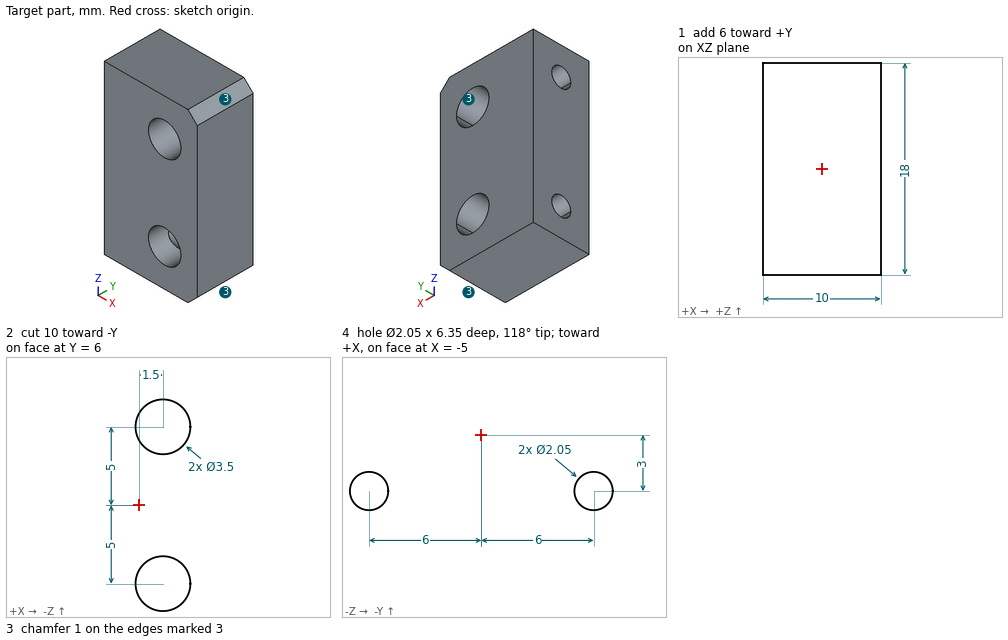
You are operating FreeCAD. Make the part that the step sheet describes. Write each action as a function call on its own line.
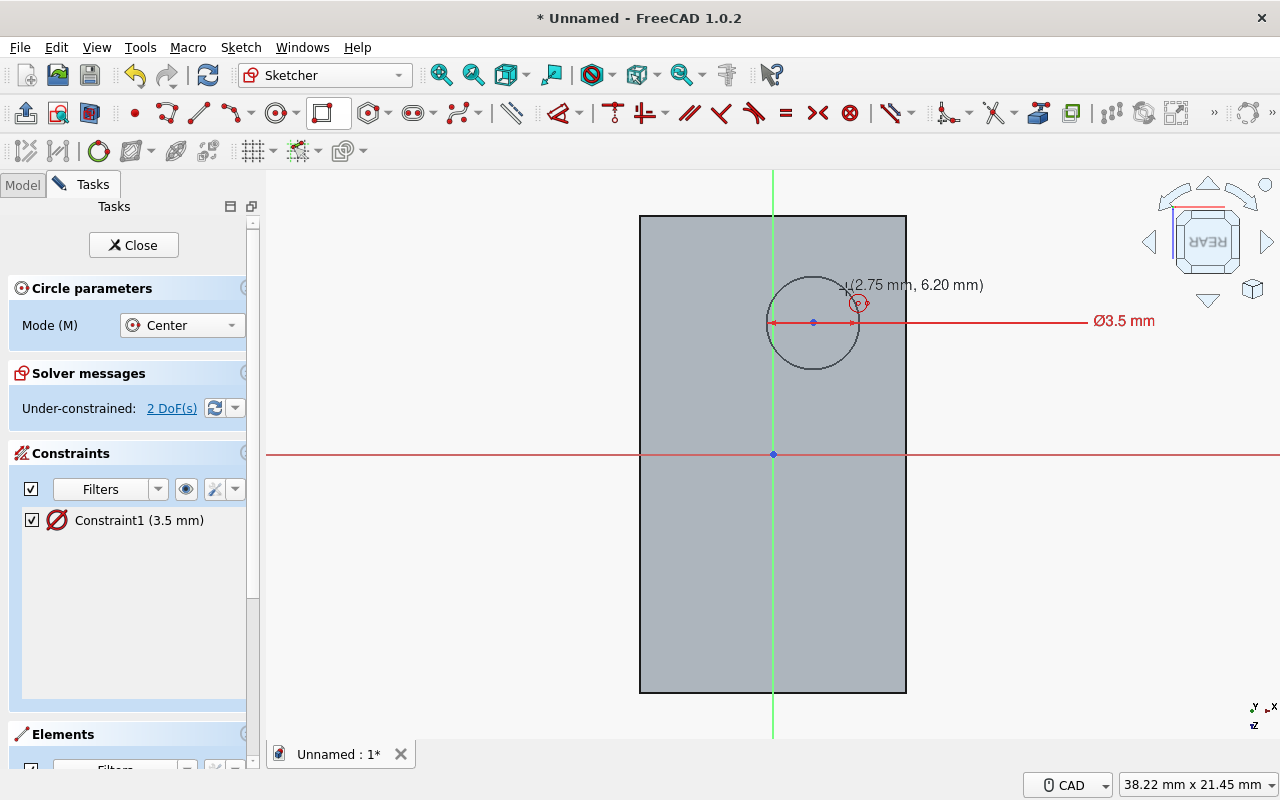
click(813, 587)
move(846, 554)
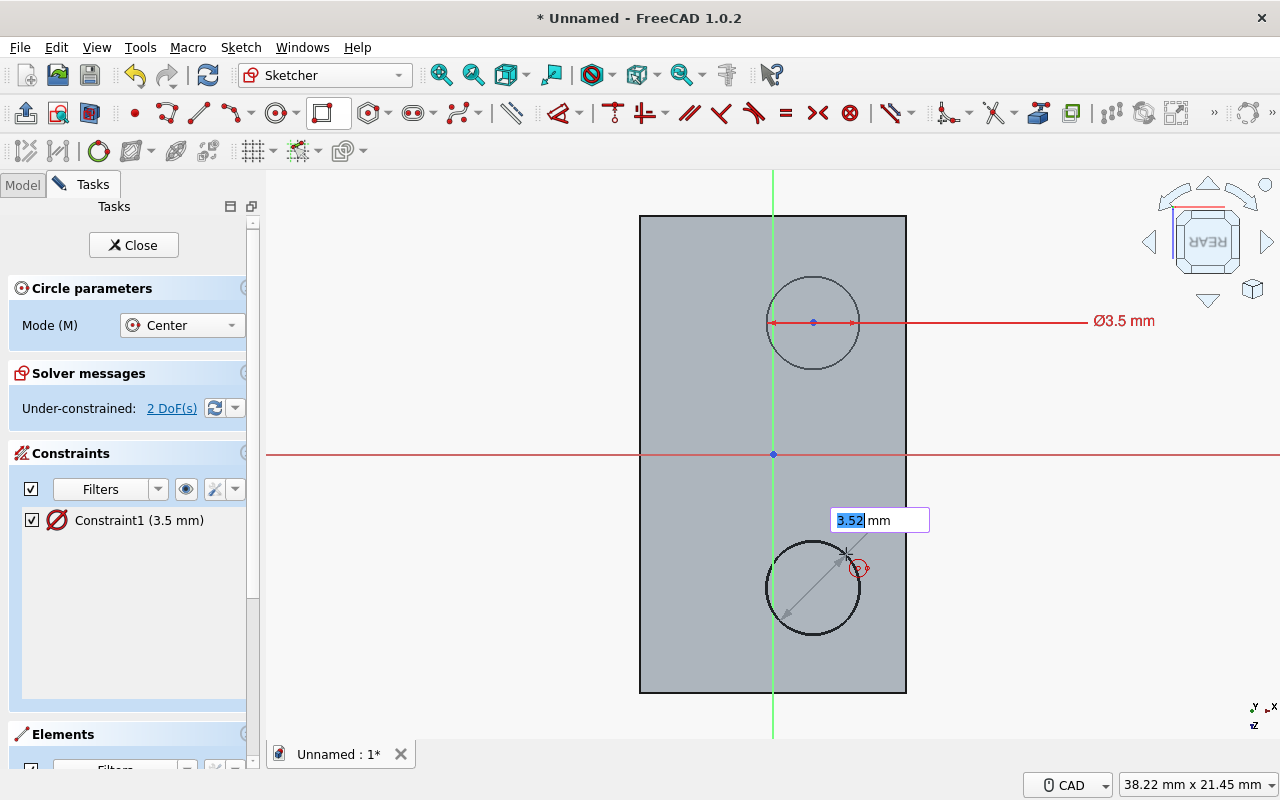
text(3.5)
key(Return)
key(Escape)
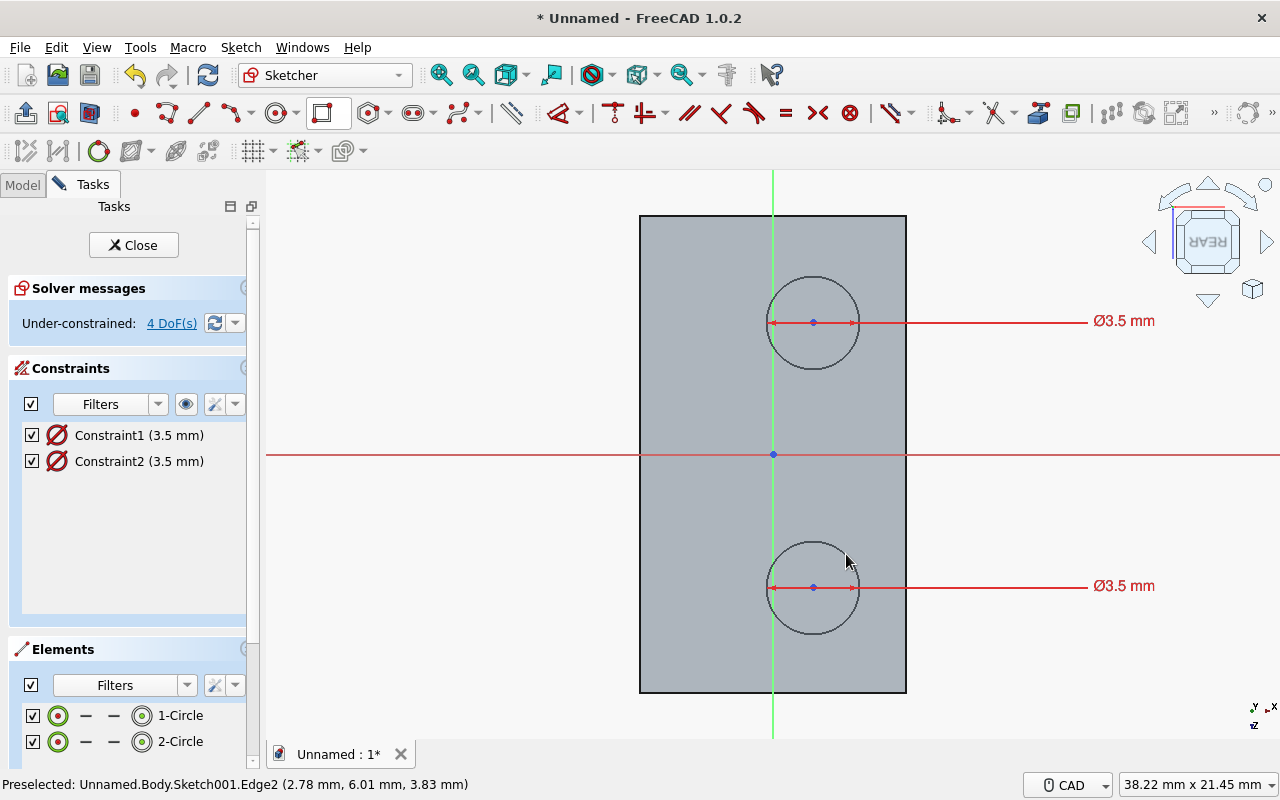
click(813, 323)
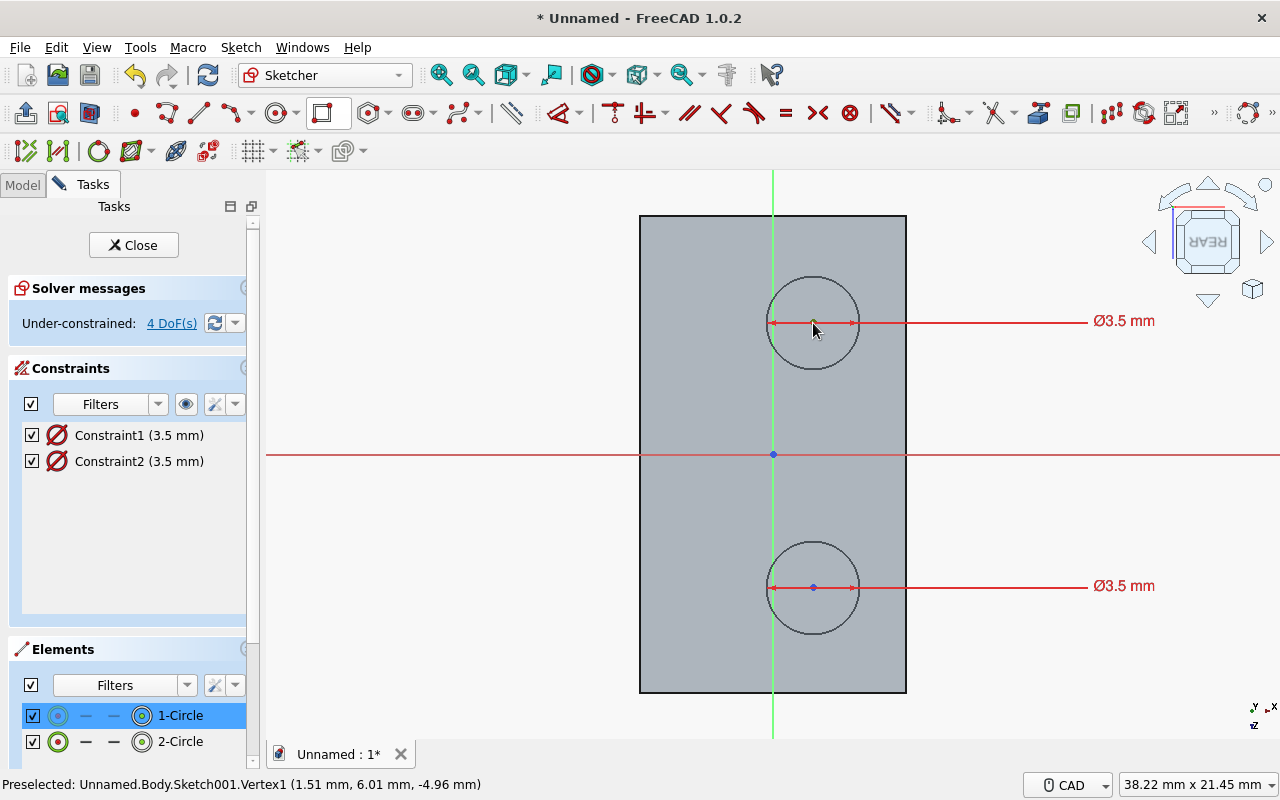
click(813, 588)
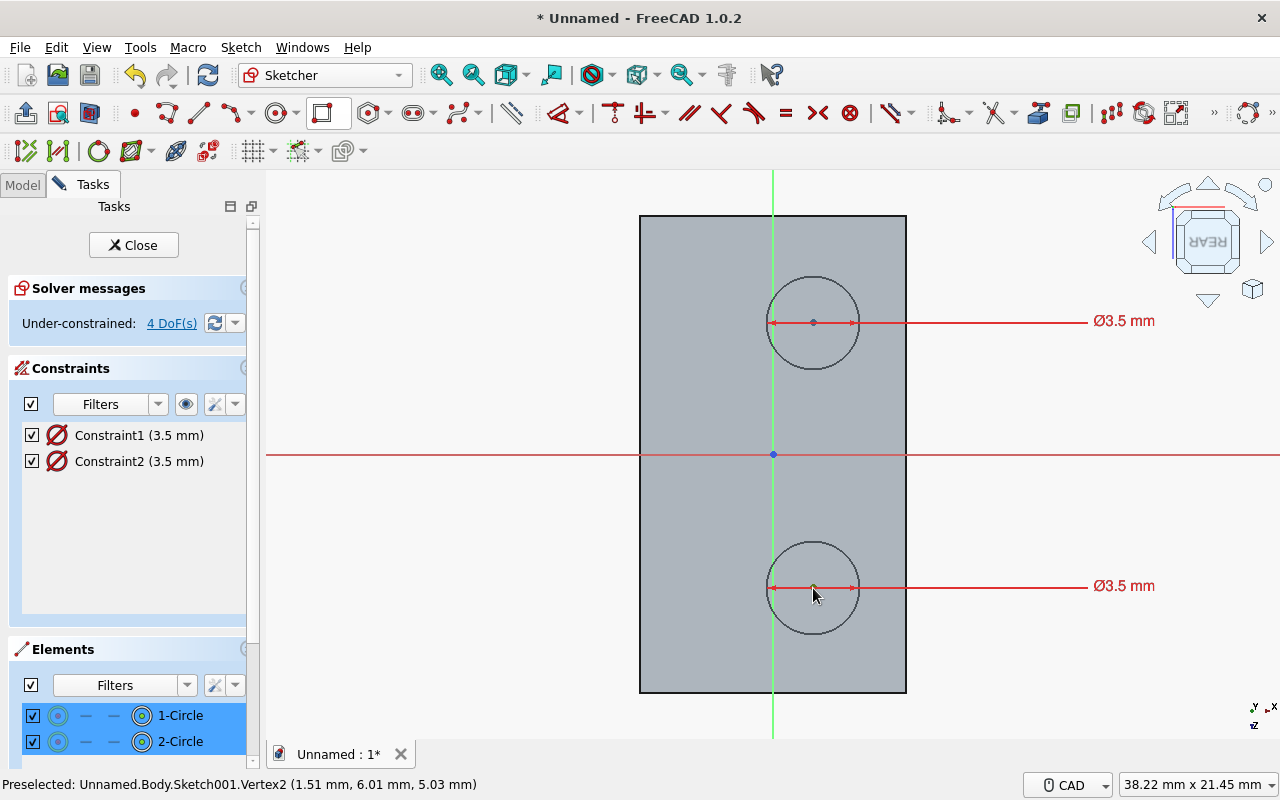
key(v)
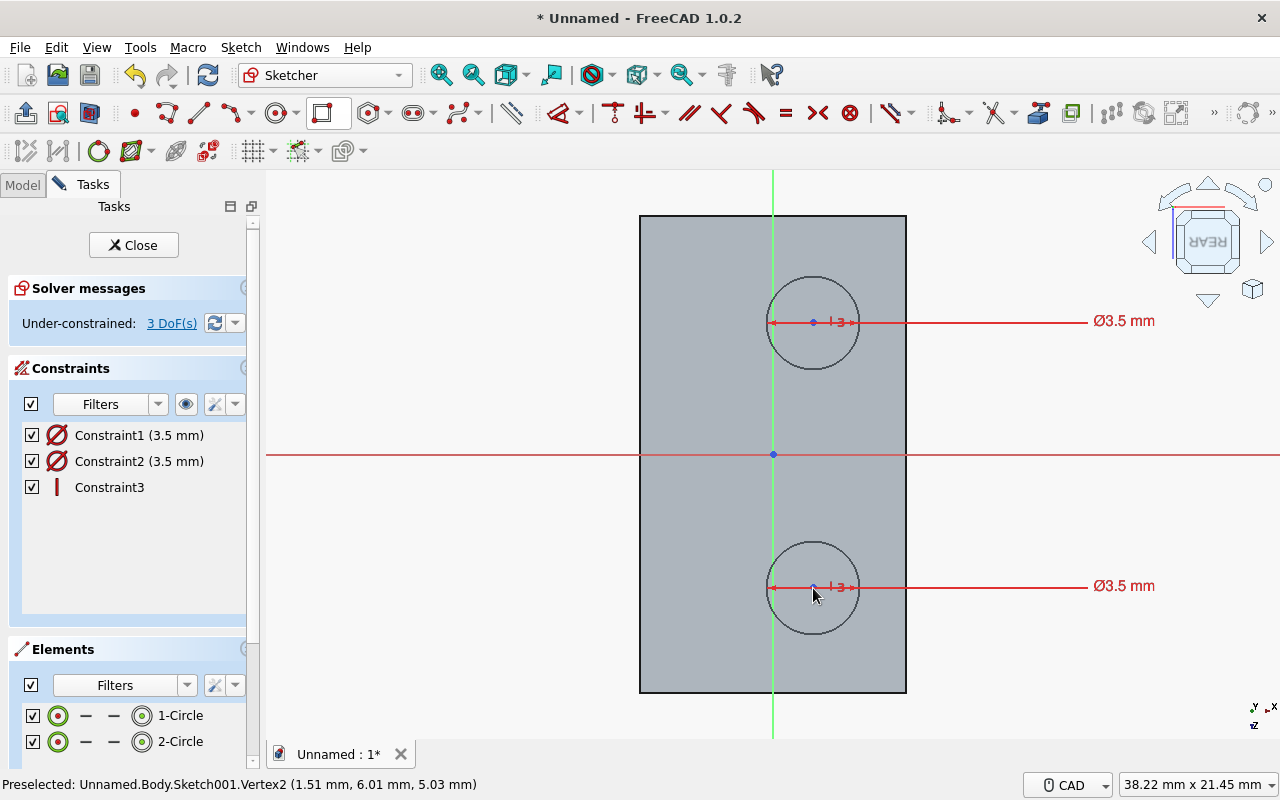
key(d)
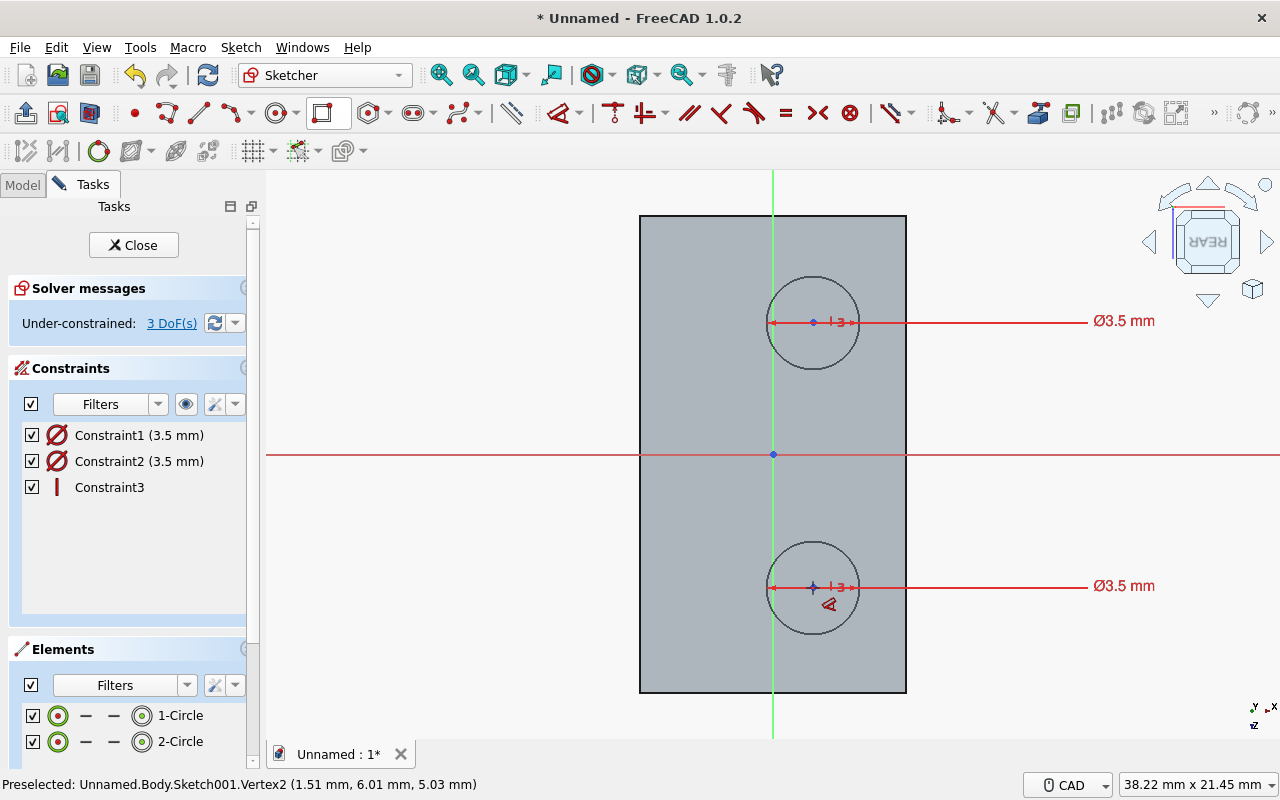
click(813, 323)
click(739, 389)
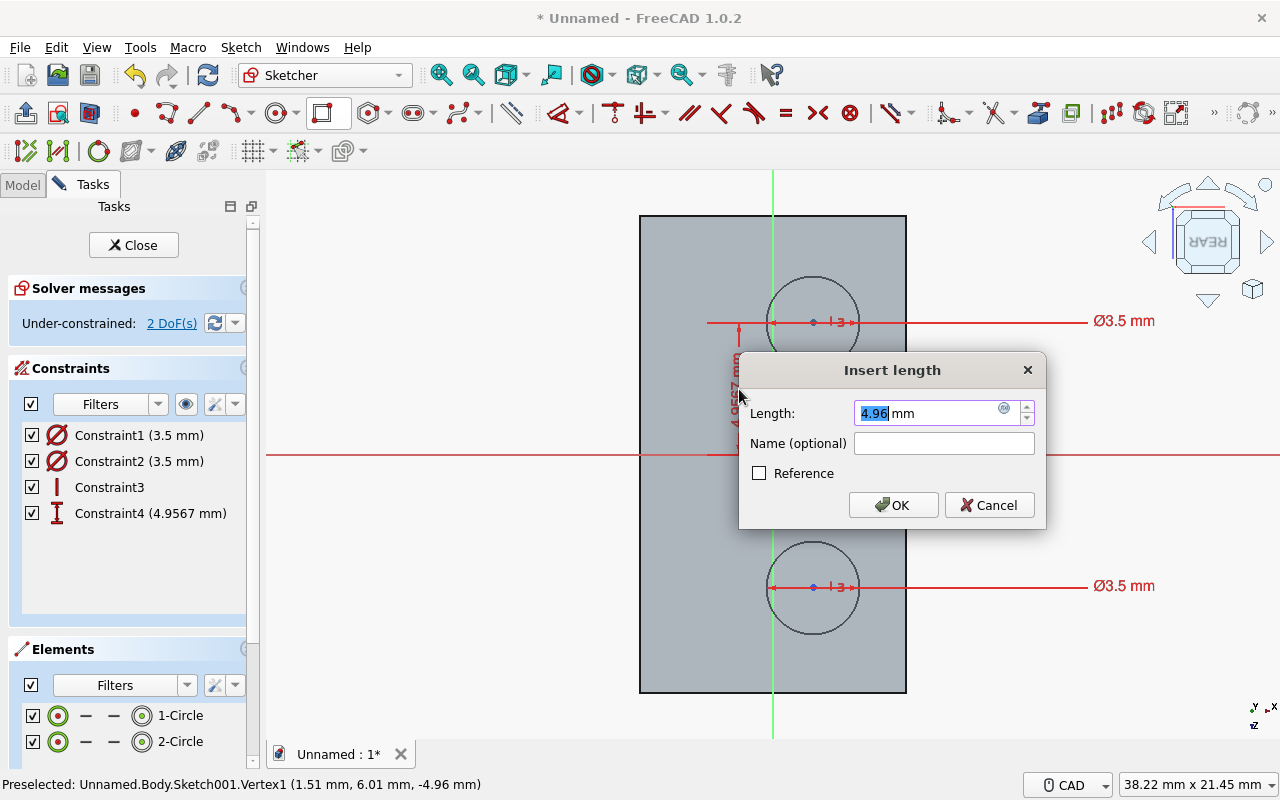
text(5)
key(Return)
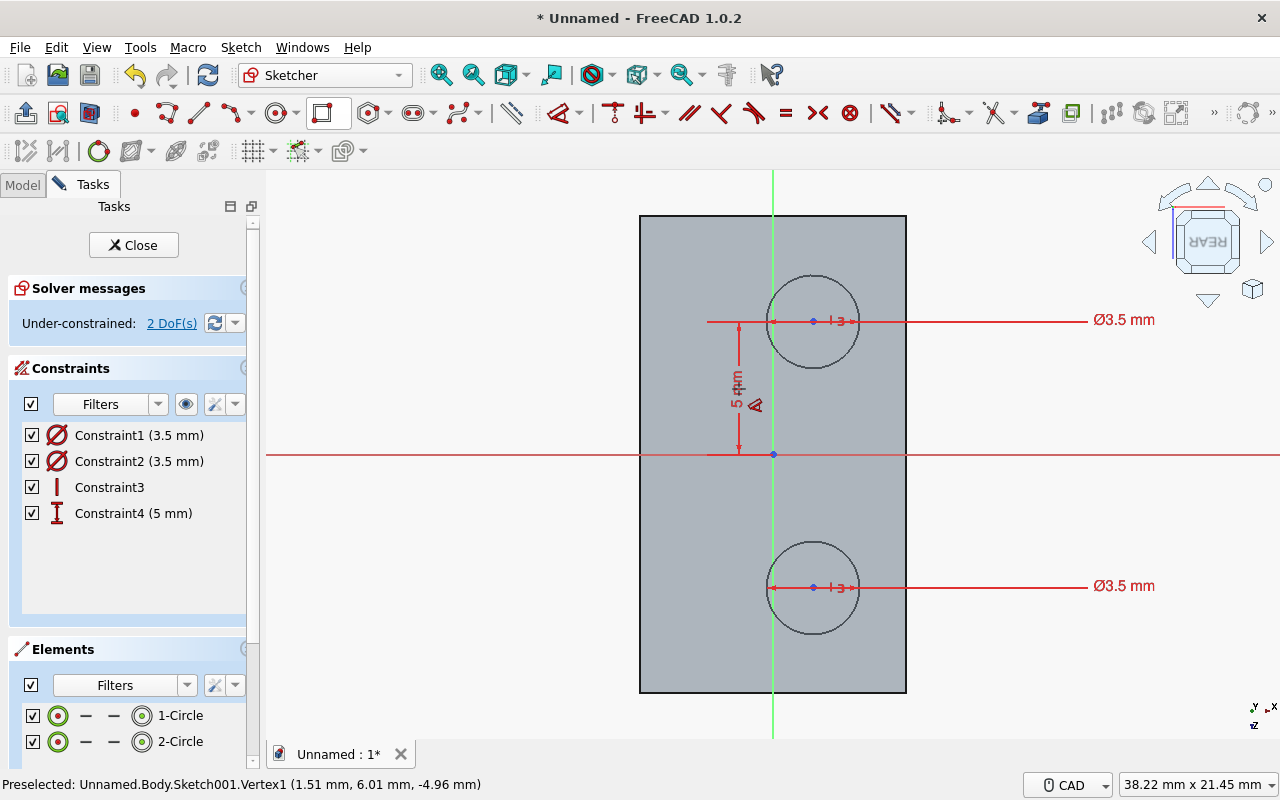
click(813, 588)
click(739, 521)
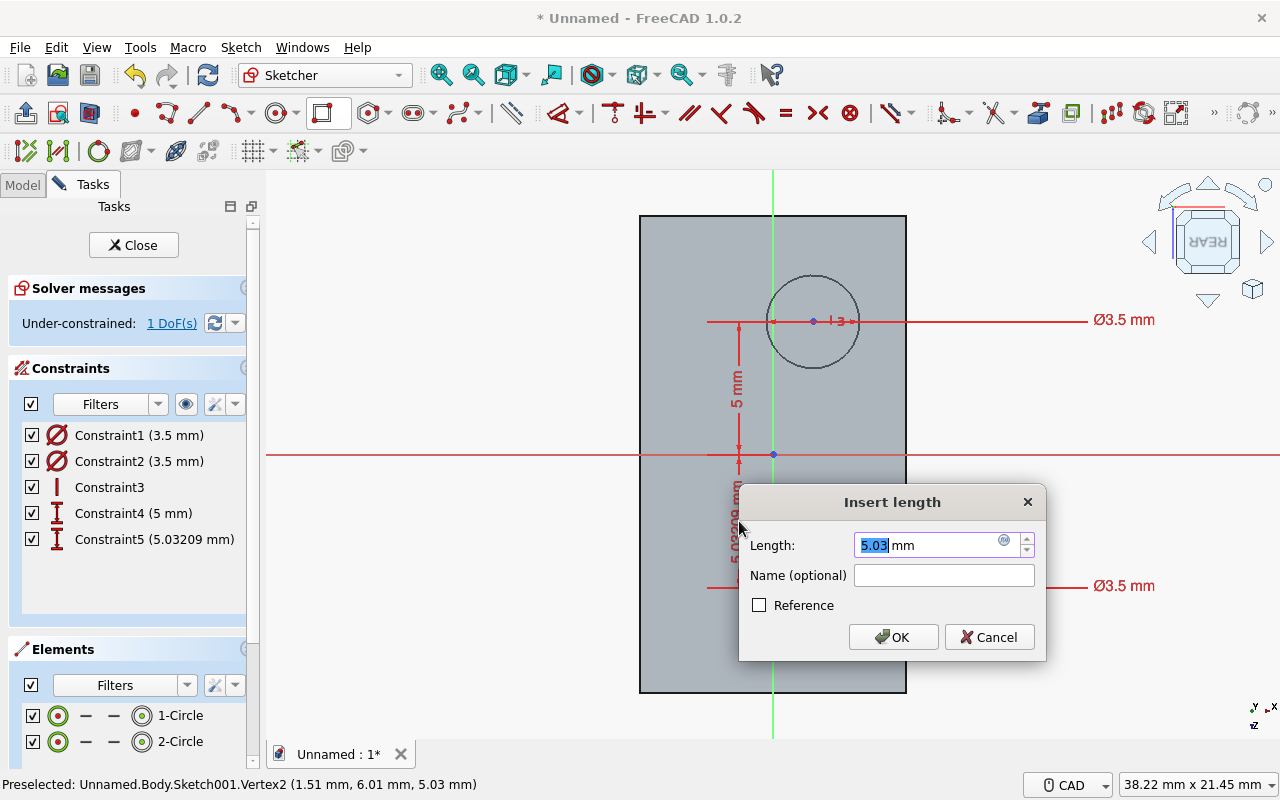
text(5)
key(Return)